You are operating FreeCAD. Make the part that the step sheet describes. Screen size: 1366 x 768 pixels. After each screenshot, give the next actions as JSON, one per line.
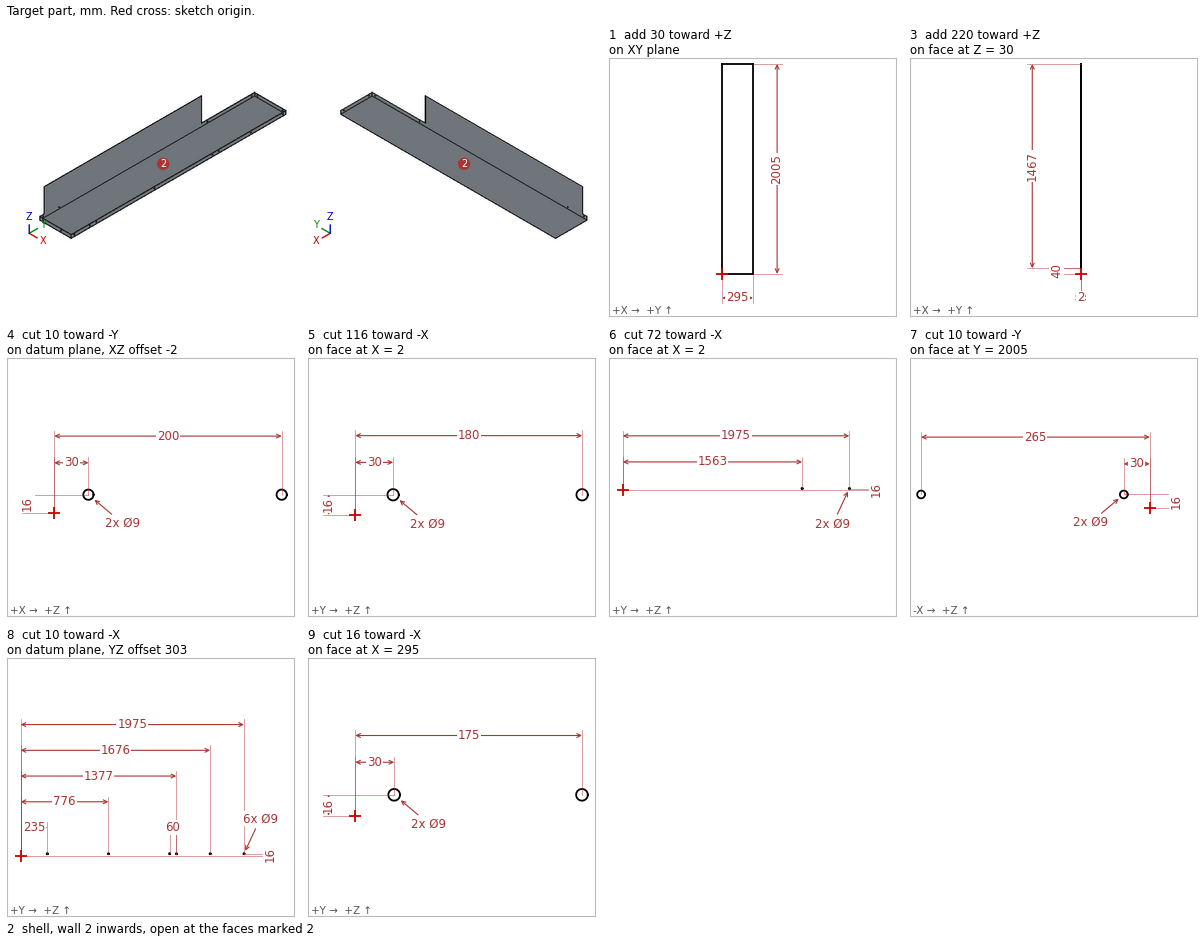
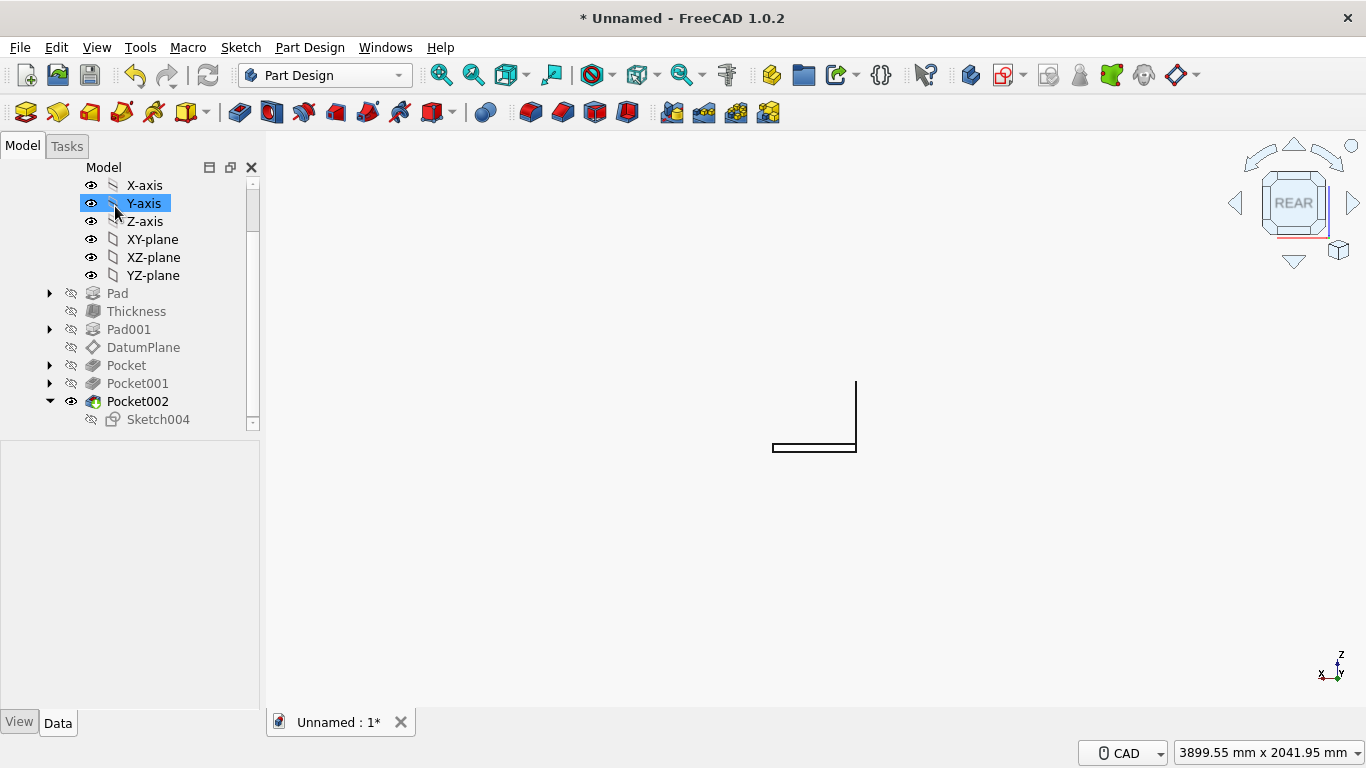
{"action": "left_click", "coordinate": [442, 76]}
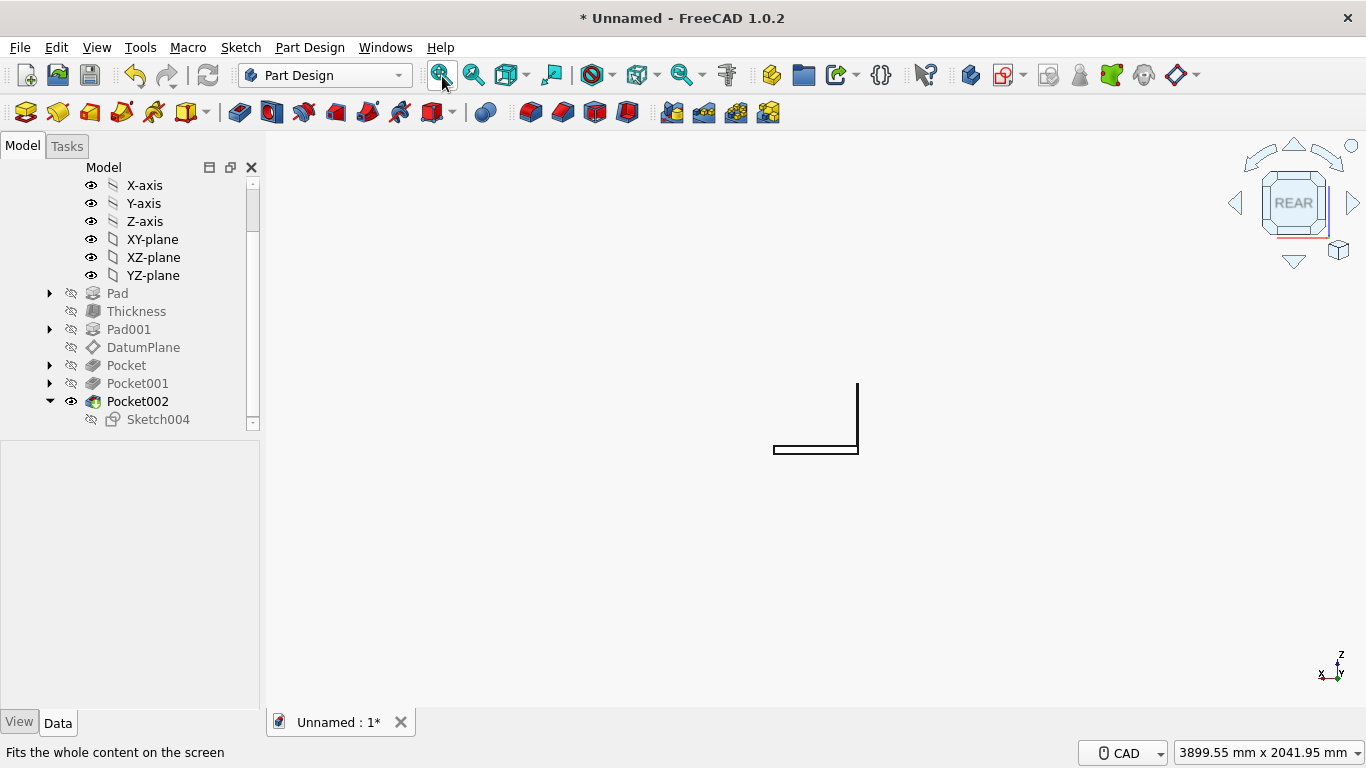
{"action": "scroll", "coordinate": [780, 449], "scroll_direction": "up", "scroll_amount": 6}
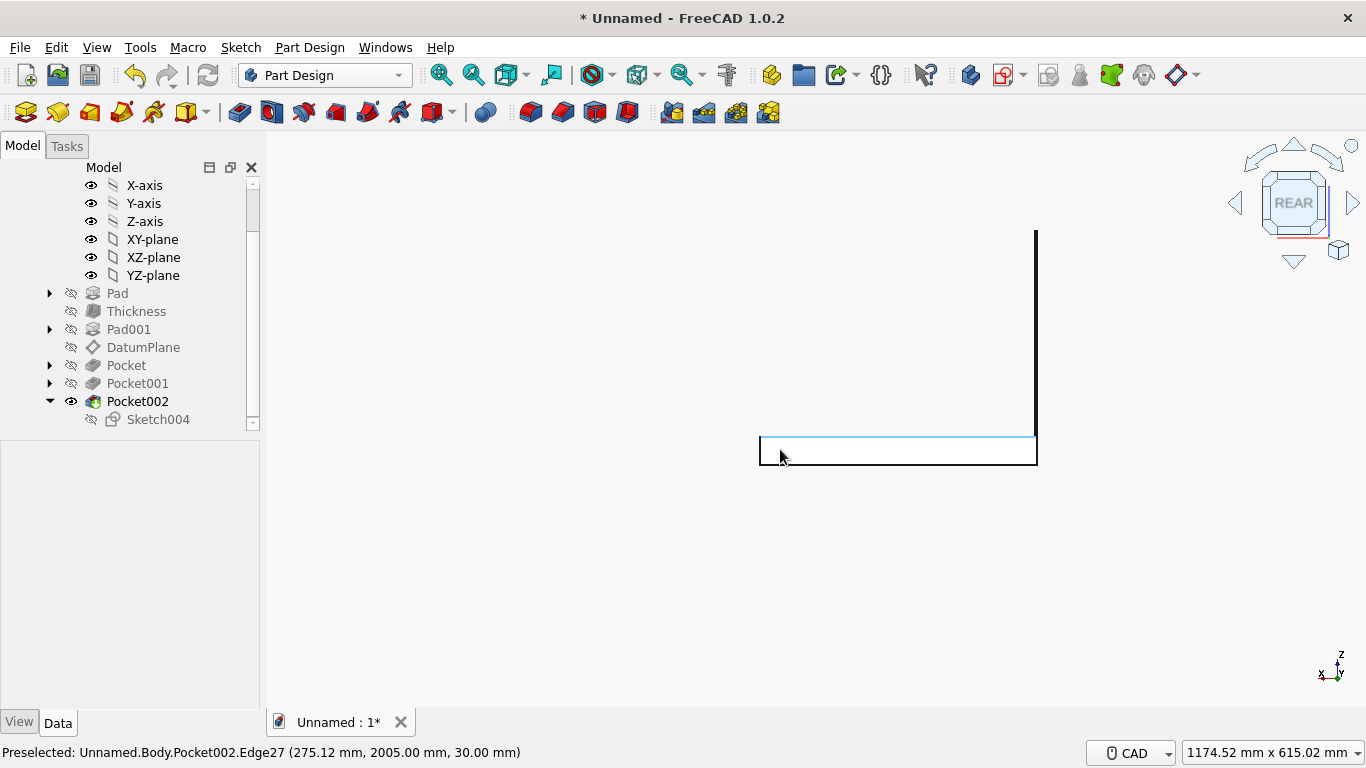
{"action": "left_click", "coordinate": [780, 450]}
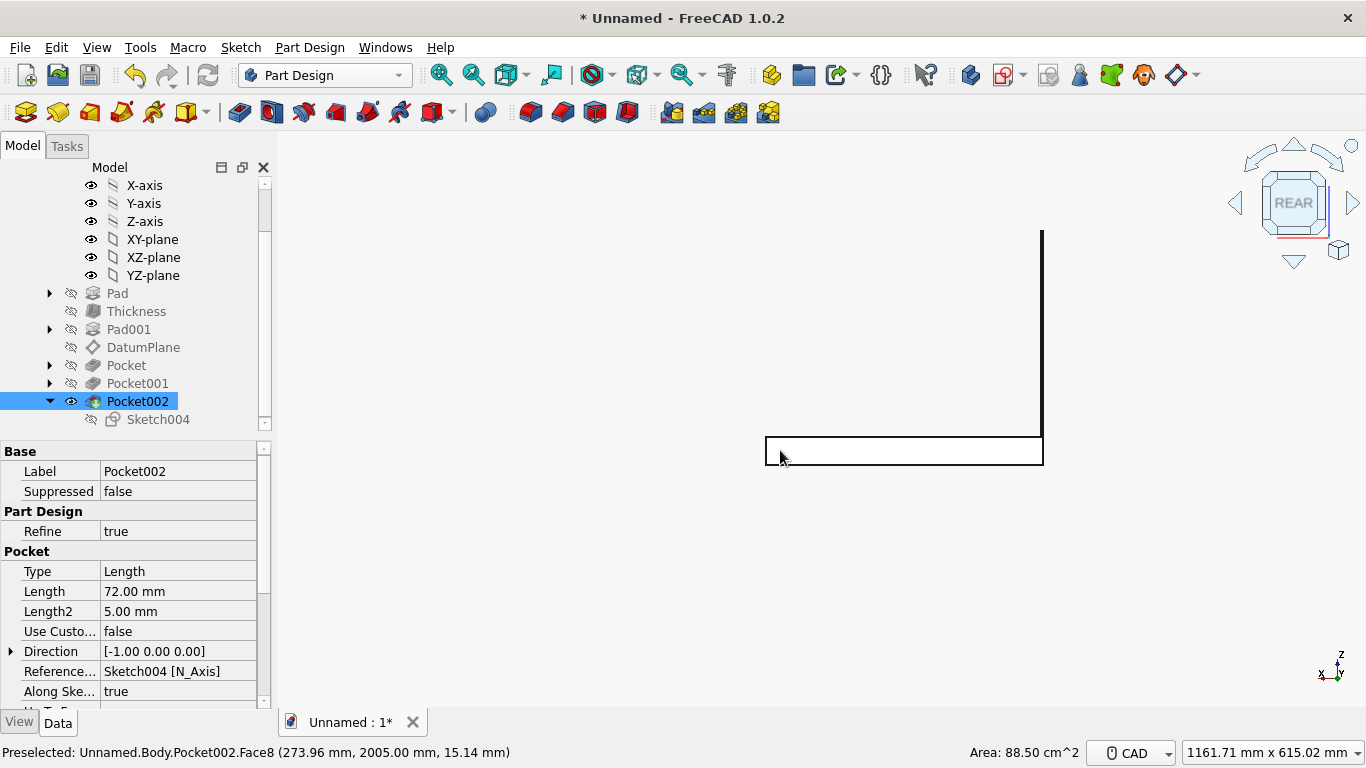
{"action": "left_click", "coordinate": [1004, 76]}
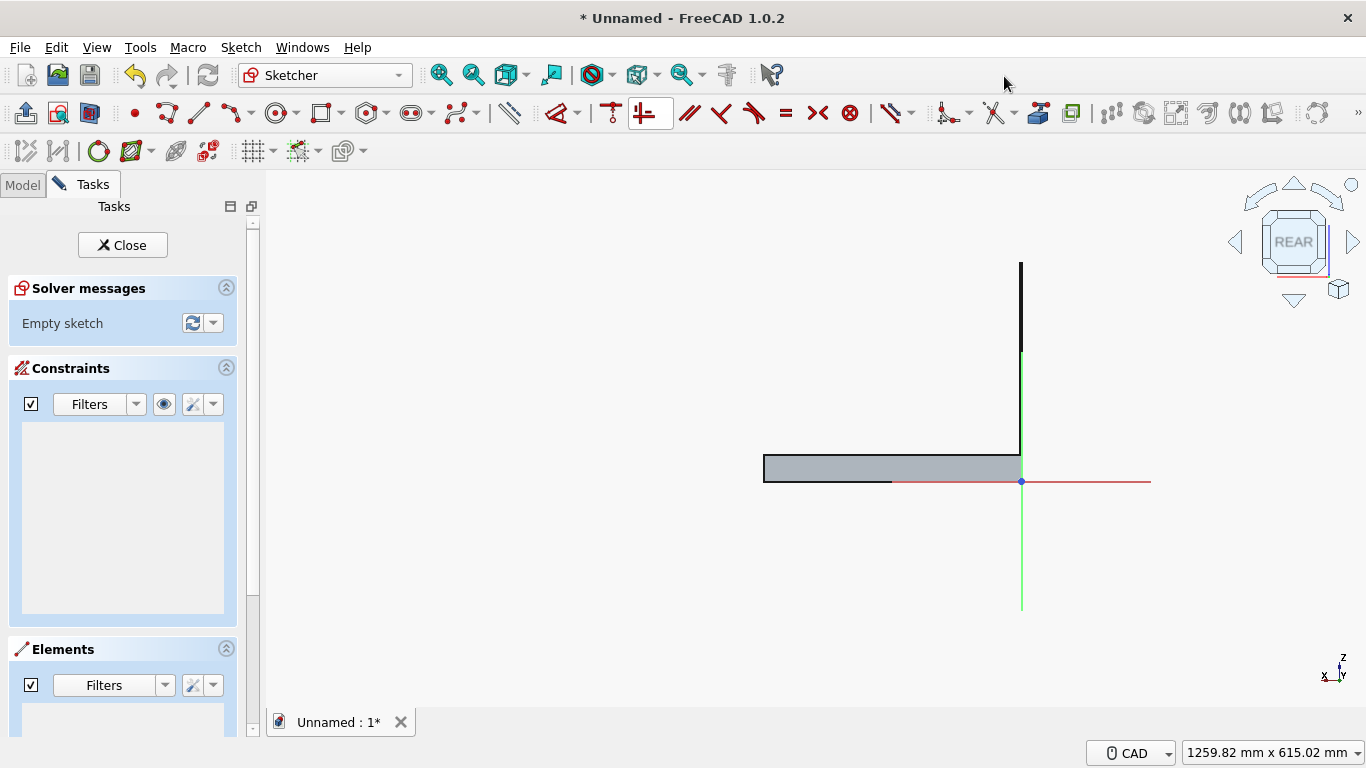
{"action": "scroll", "coordinate": [995, 492], "scroll_direction": "up", "scroll_amount": 5}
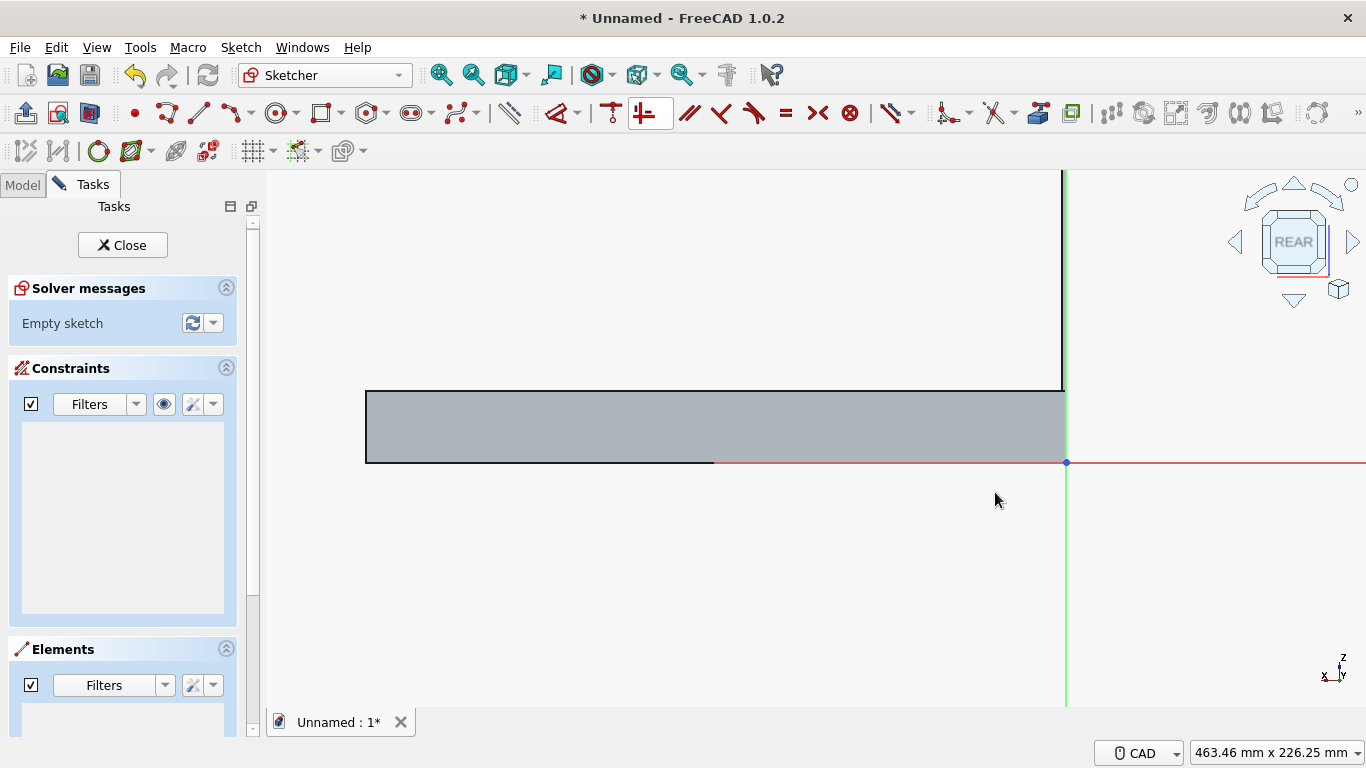
{"action": "left_click", "coordinate": [276, 114]}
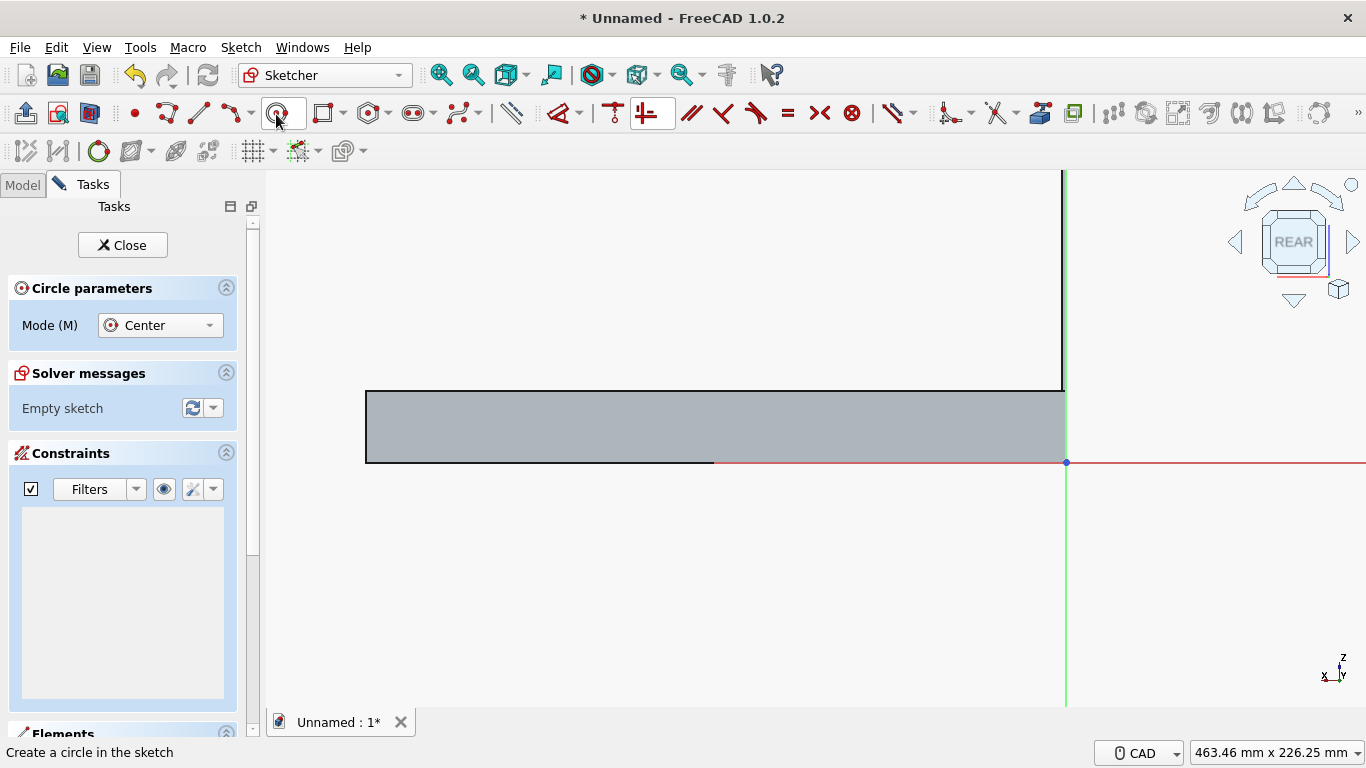
{"action": "scroll", "coordinate": [995, 425], "scroll_direction": "up", "scroll_amount": 4}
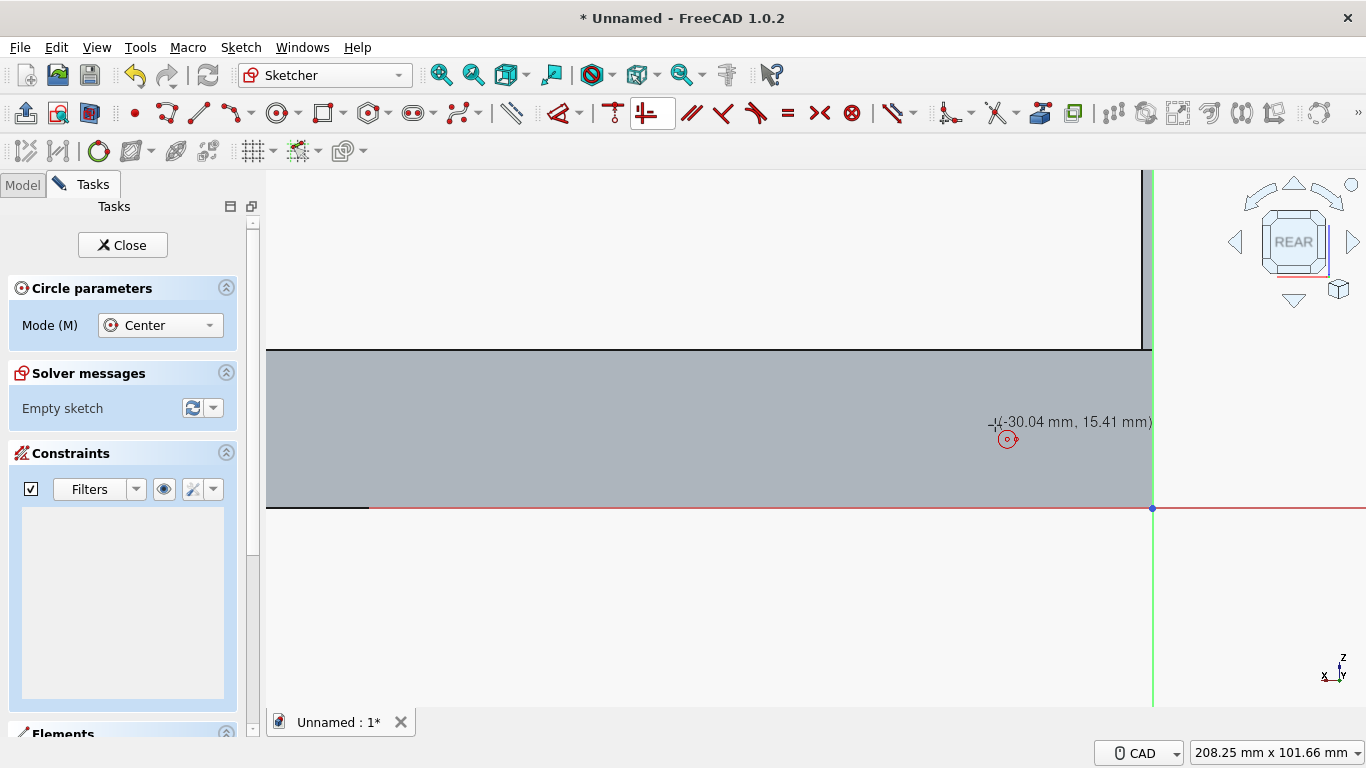
{"action": "left_click", "coordinate": [994, 424]}
{"action": "left_click", "coordinate": [1011, 407]}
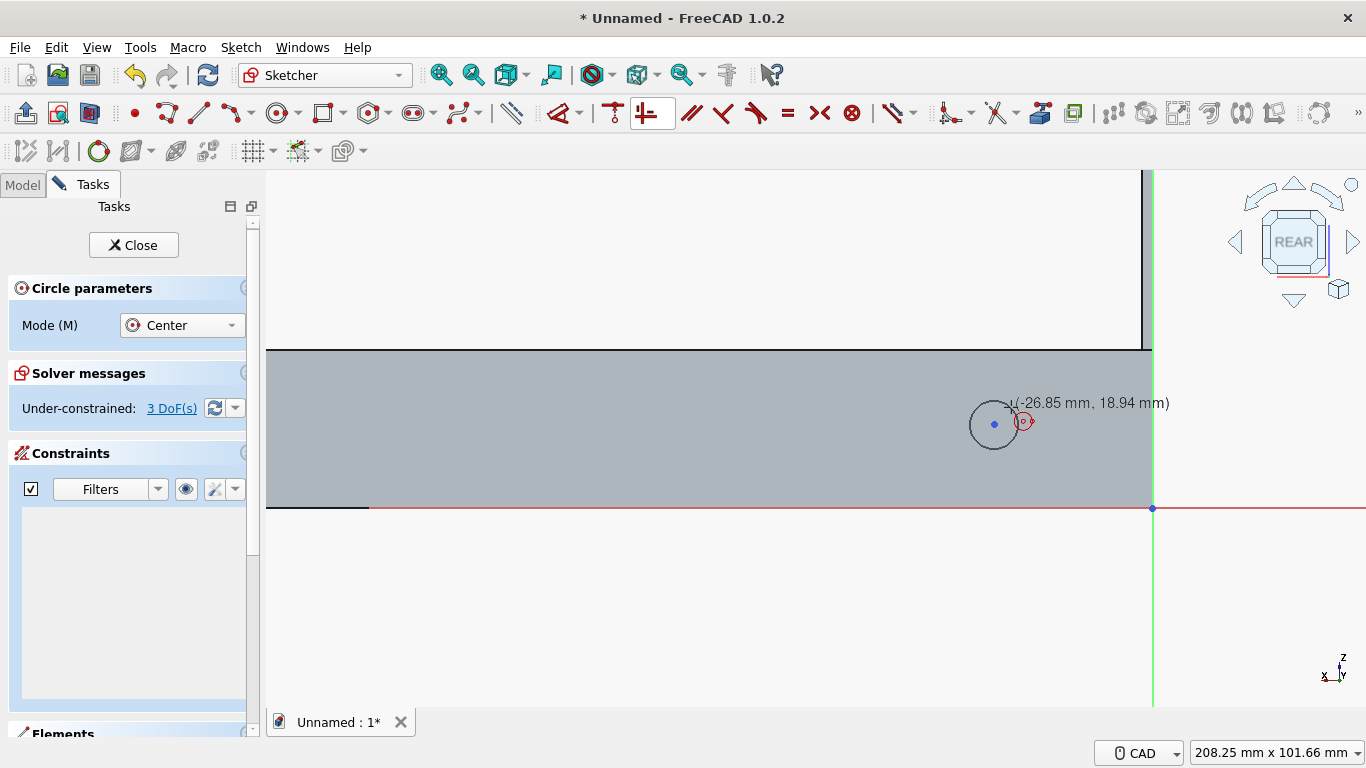
{"action": "scroll", "coordinate": [998, 426], "scroll_direction": "down", "scroll_amount": 4}